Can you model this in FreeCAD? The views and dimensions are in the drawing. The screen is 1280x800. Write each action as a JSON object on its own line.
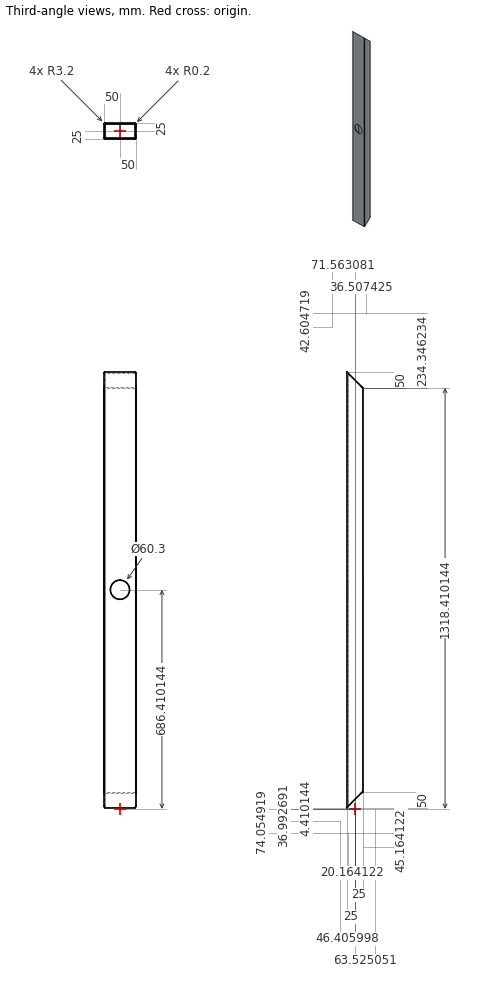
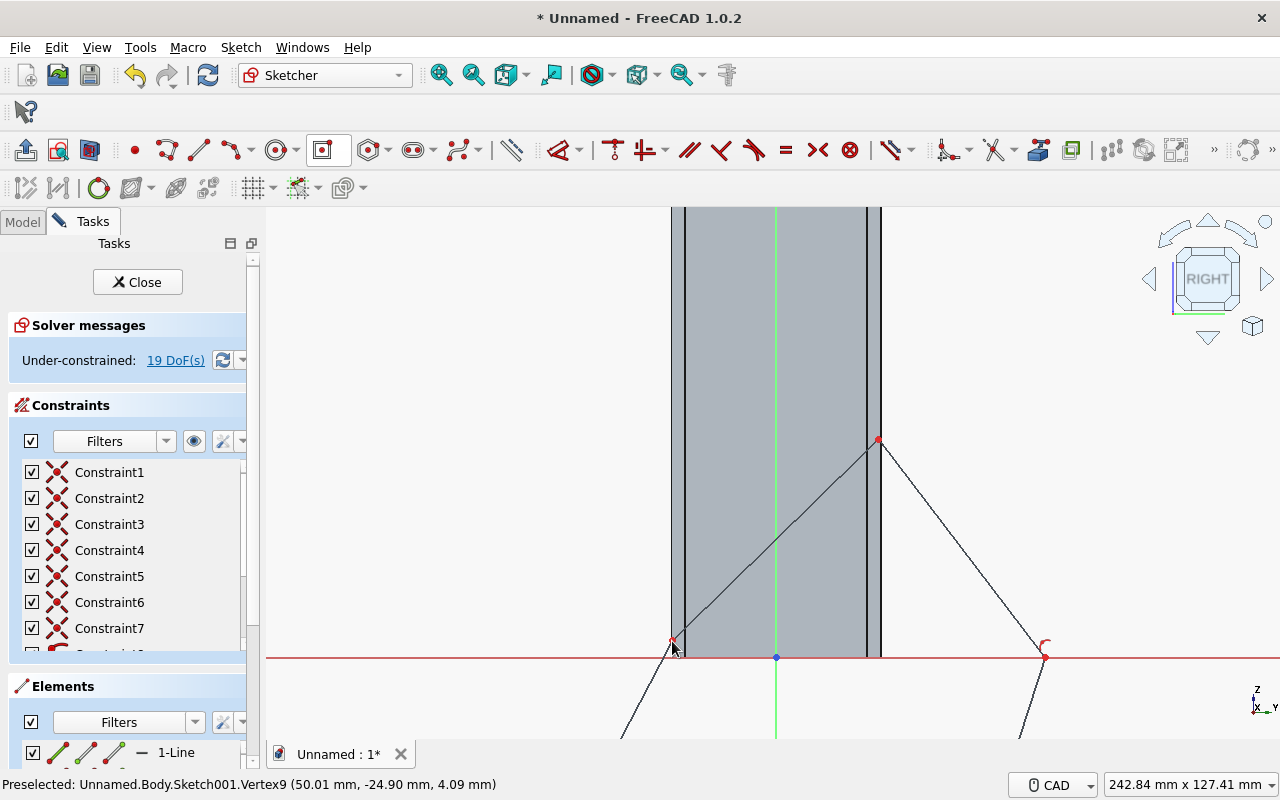
{"action": "left_click", "coordinate": [558, 150]}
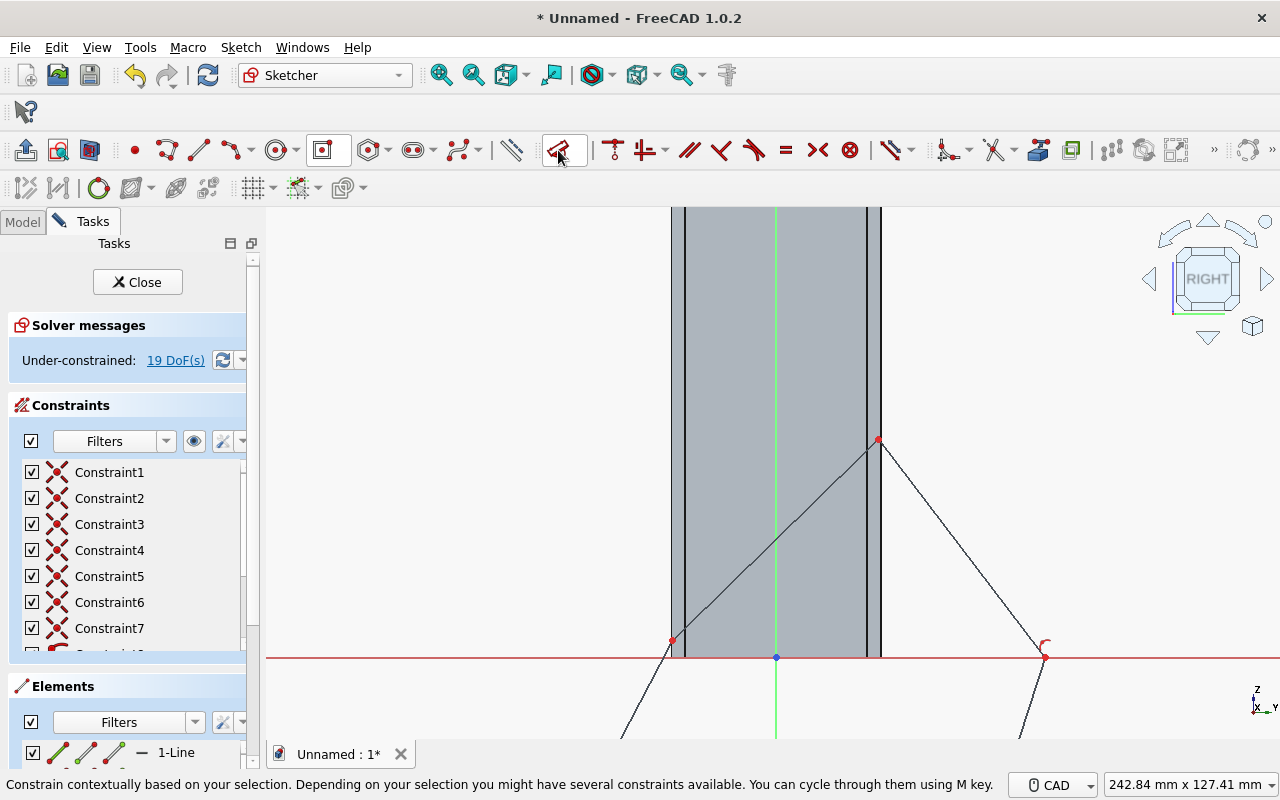
{"action": "scroll", "coordinate": [702, 620], "scroll_direction": "down", "scroll_amount": 15}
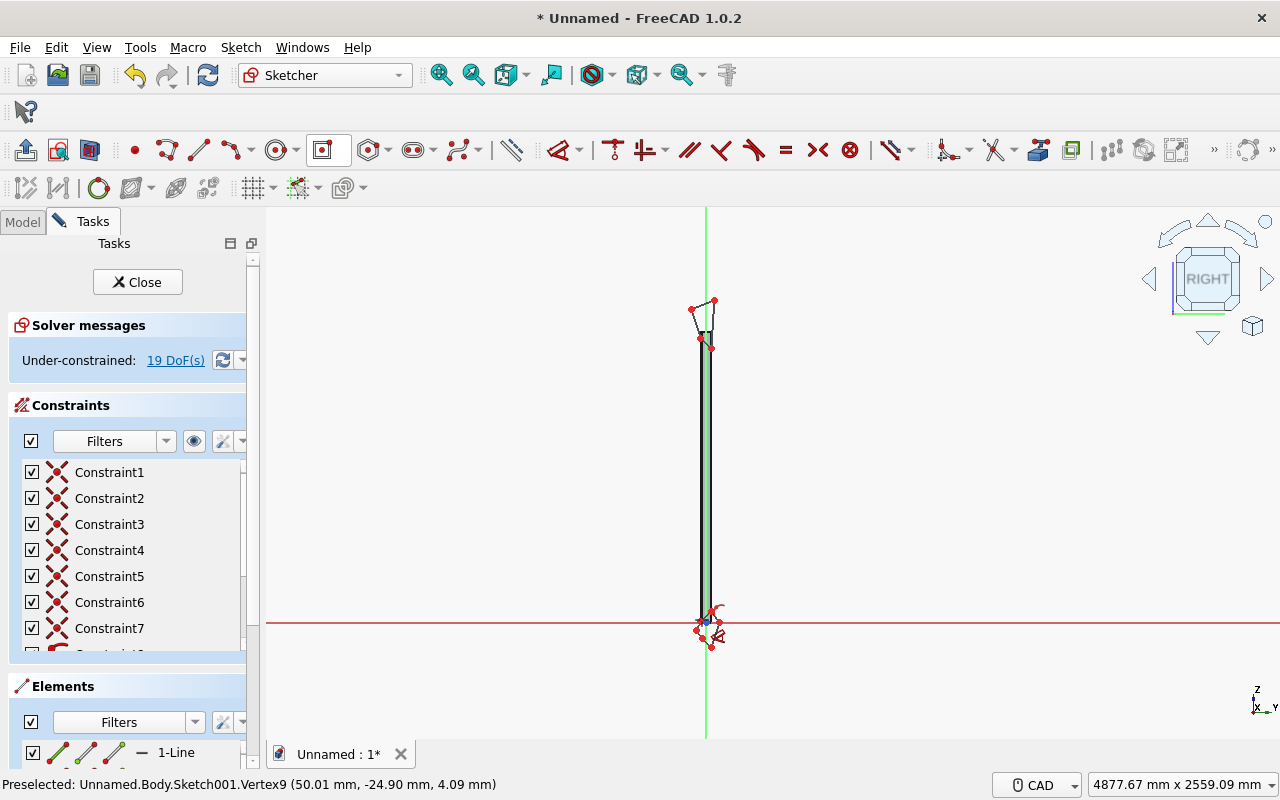
{"action": "scroll", "coordinate": [711, 349], "scroll_direction": "up", "scroll_amount": 11}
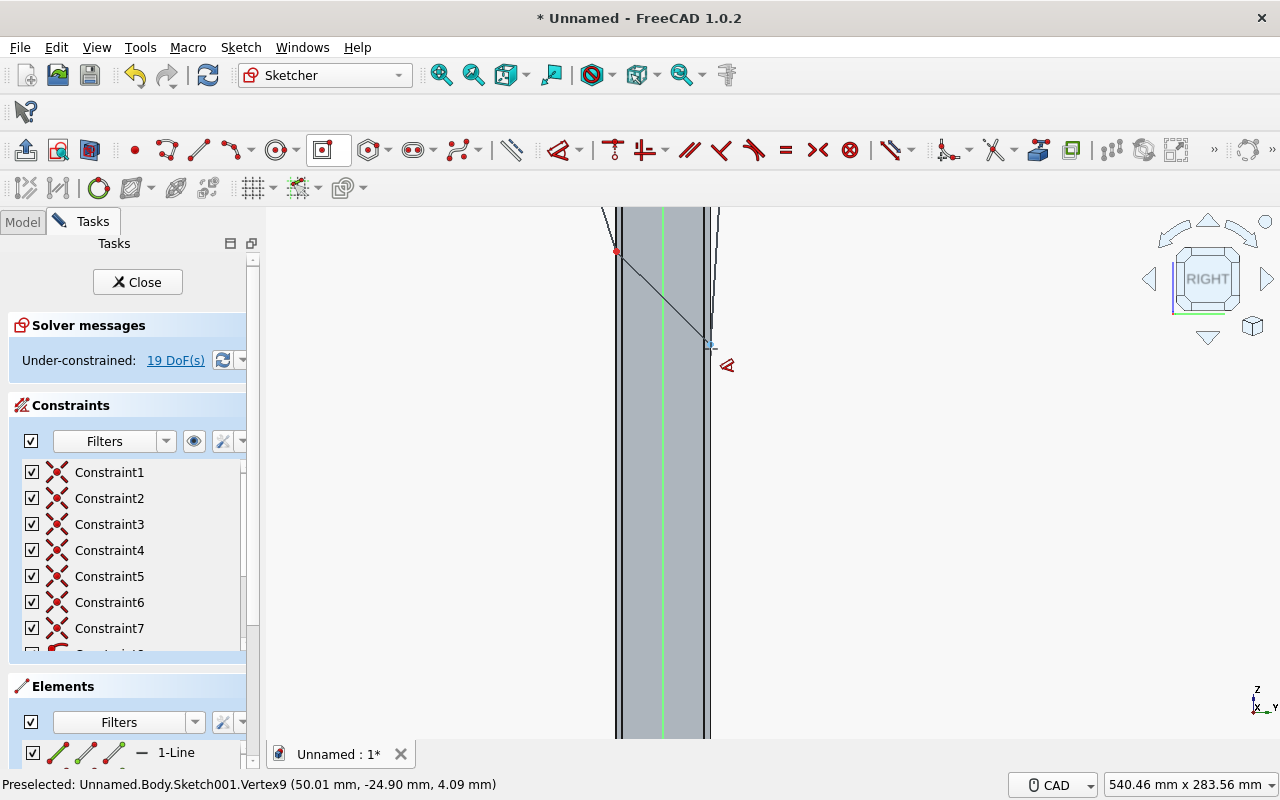
{"action": "left_click", "coordinate": [711, 345]}
{"action": "left_click", "coordinate": [698, 311]}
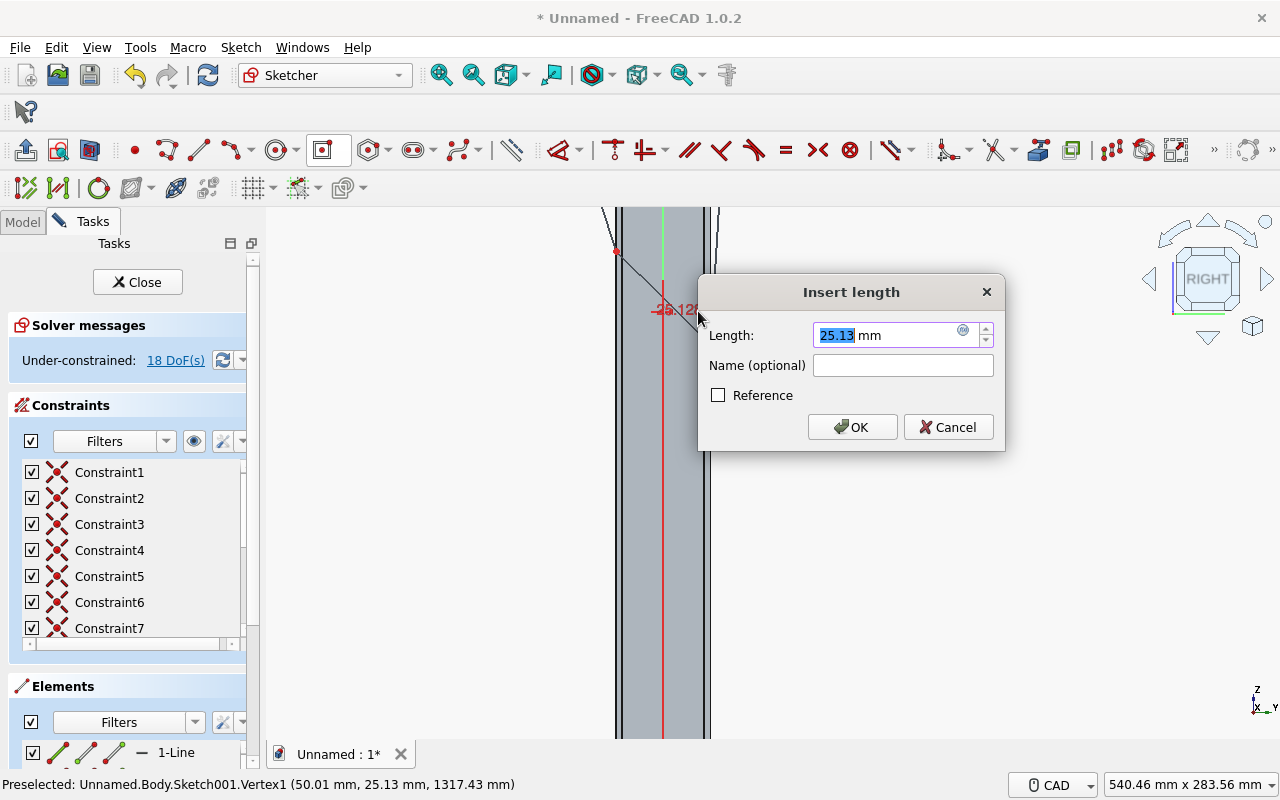
{"action": "type", "text": "25"}
{"action": "key", "text": "Return"}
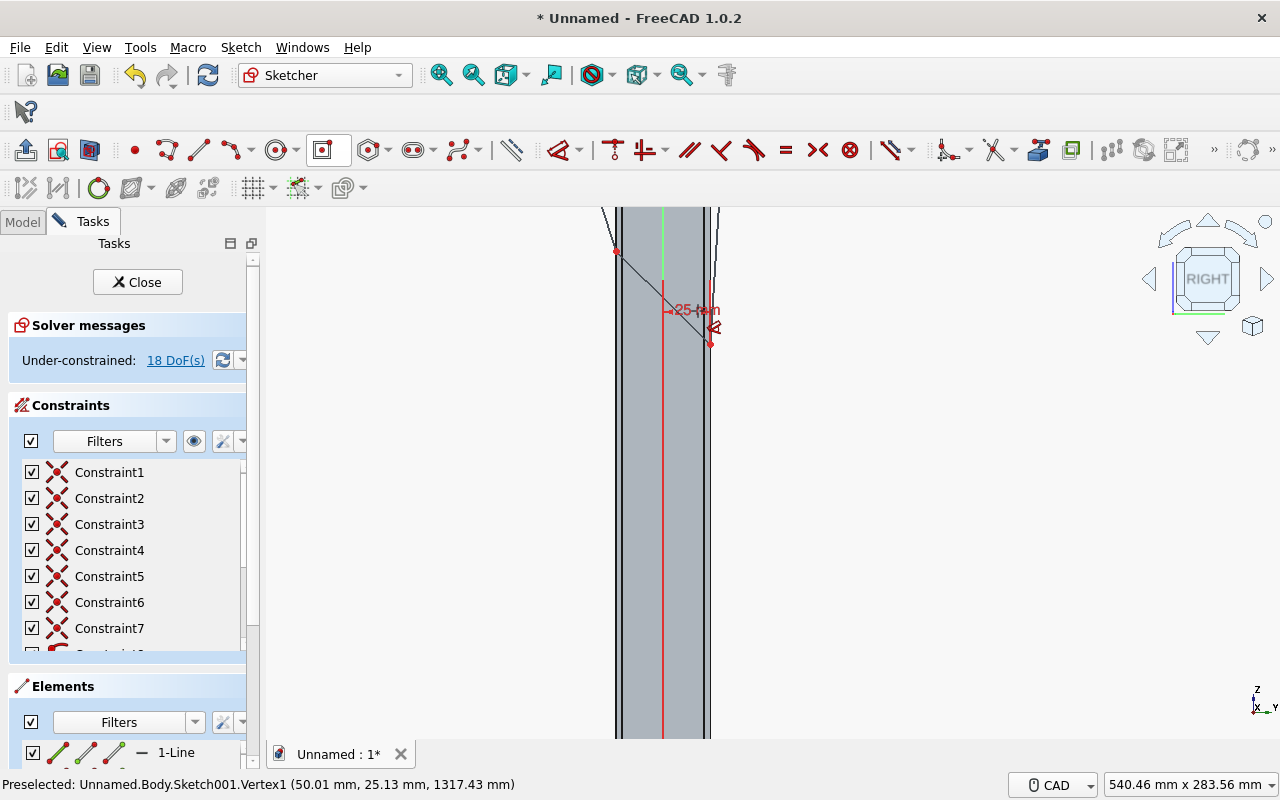
{"action": "left_click", "coordinate": [616, 252]}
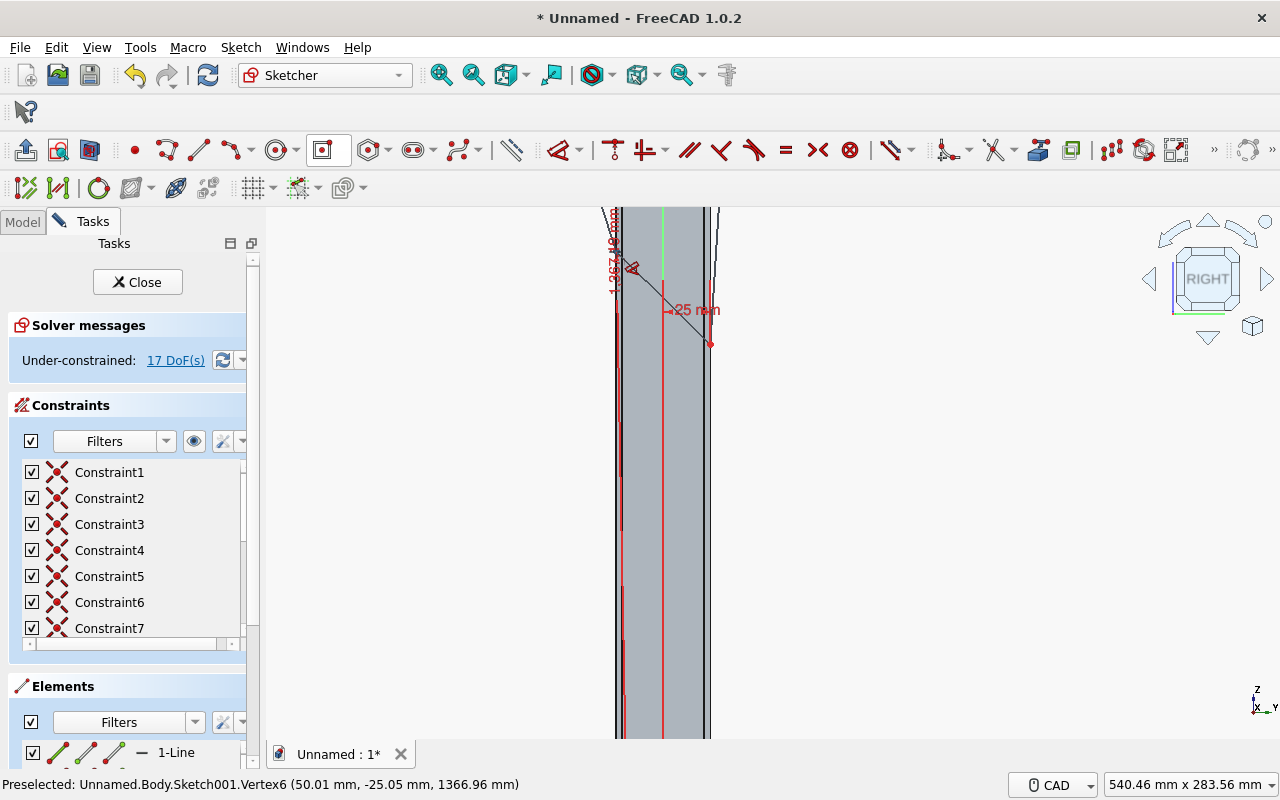
{"action": "key", "text": "Escape"}
{"action": "key", "text": "Escape"}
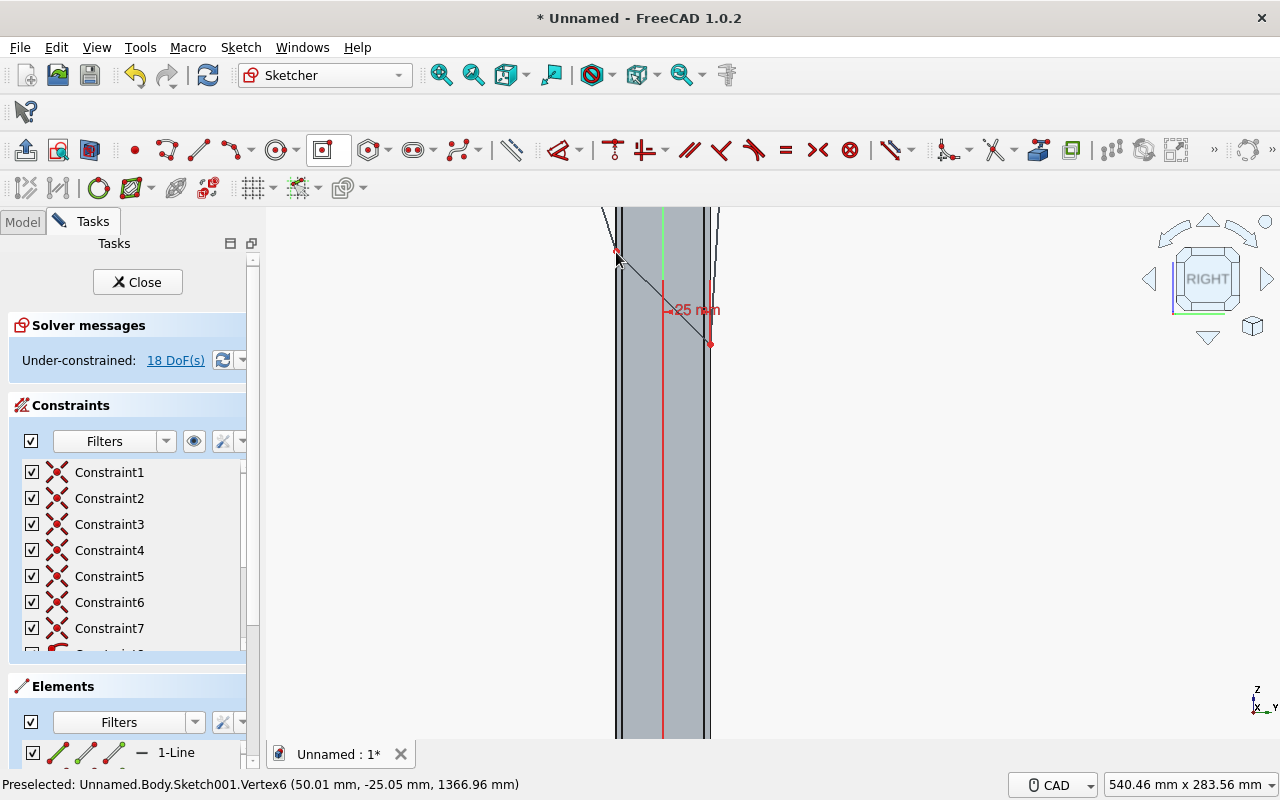
{"action": "left_click", "coordinate": [616, 252]}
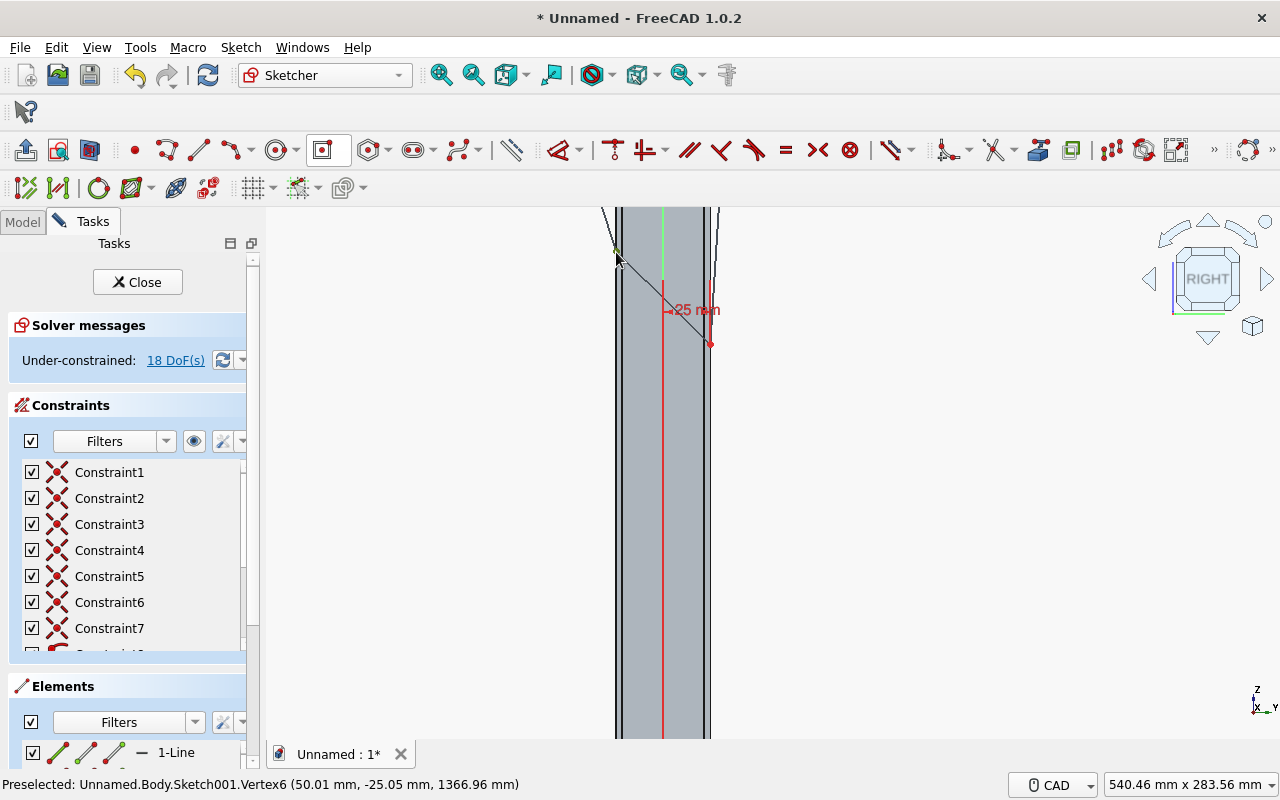
{"action": "key", "text": "l"}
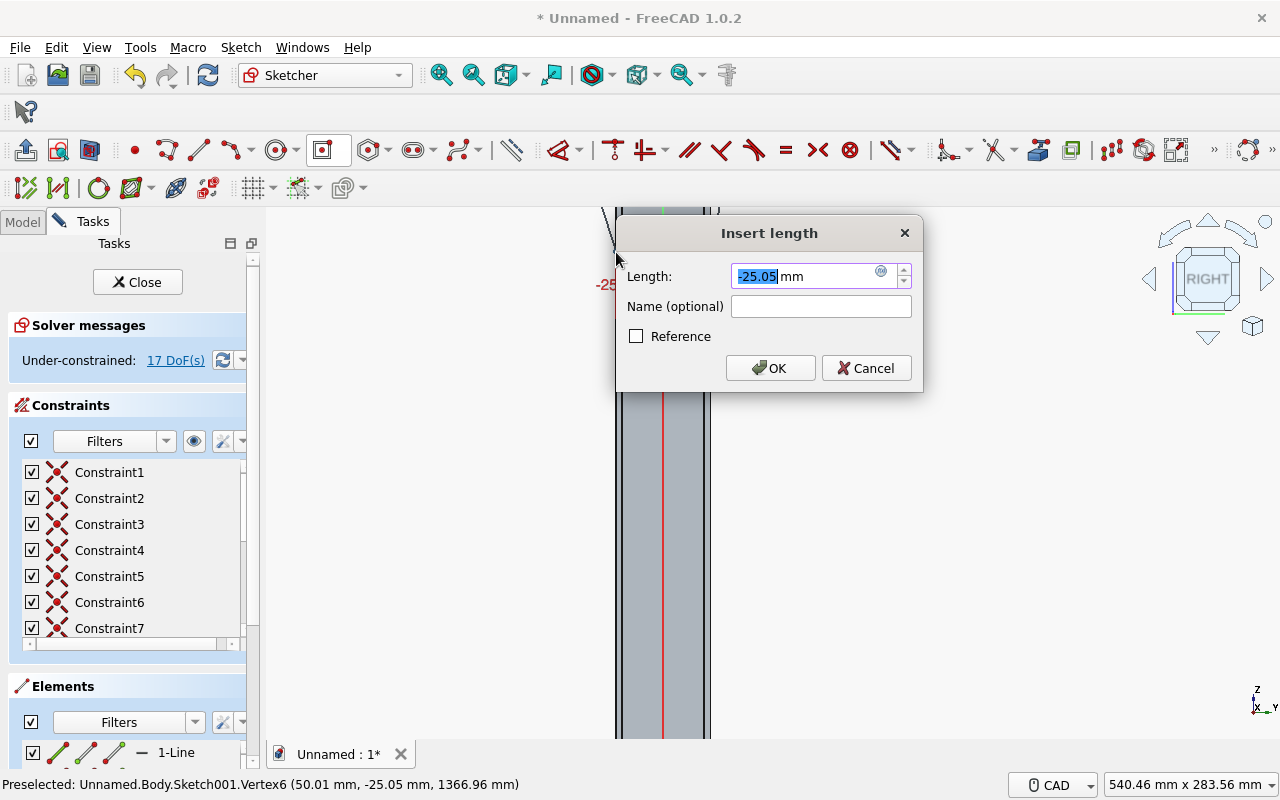
{"action": "type", "text": "-25"}
{"action": "key", "text": "Return"}